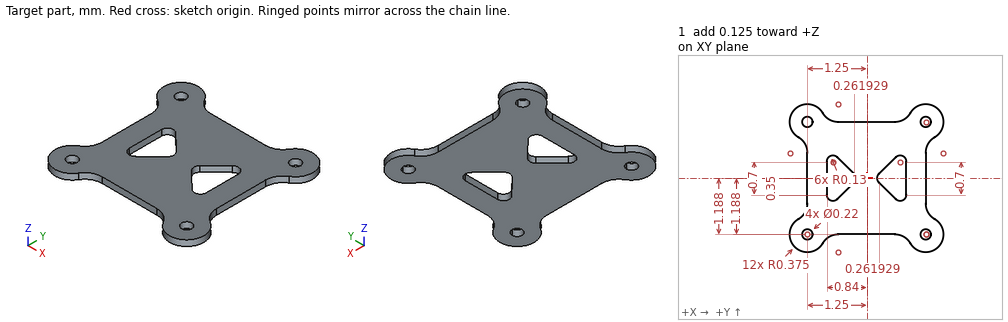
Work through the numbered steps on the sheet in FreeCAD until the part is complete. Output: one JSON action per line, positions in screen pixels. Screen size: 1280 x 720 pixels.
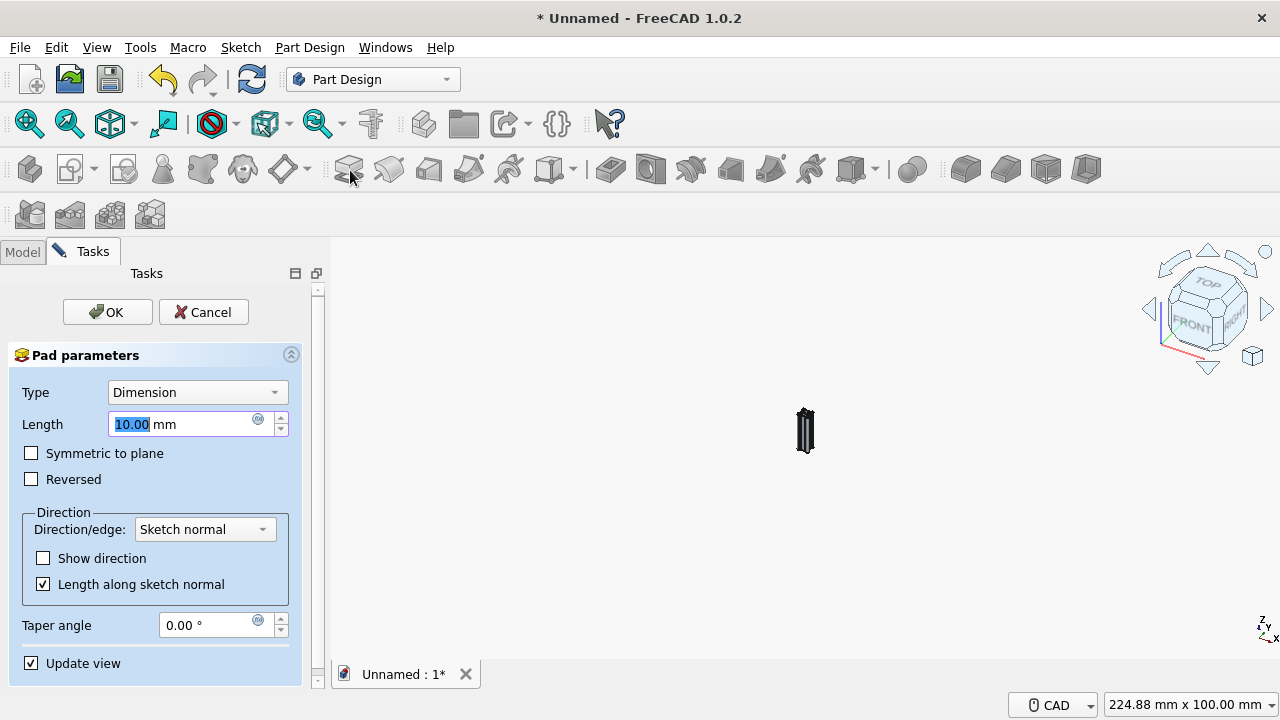
{"action": "type", "text": "0.125"}
{"action": "key", "text": "Tab"}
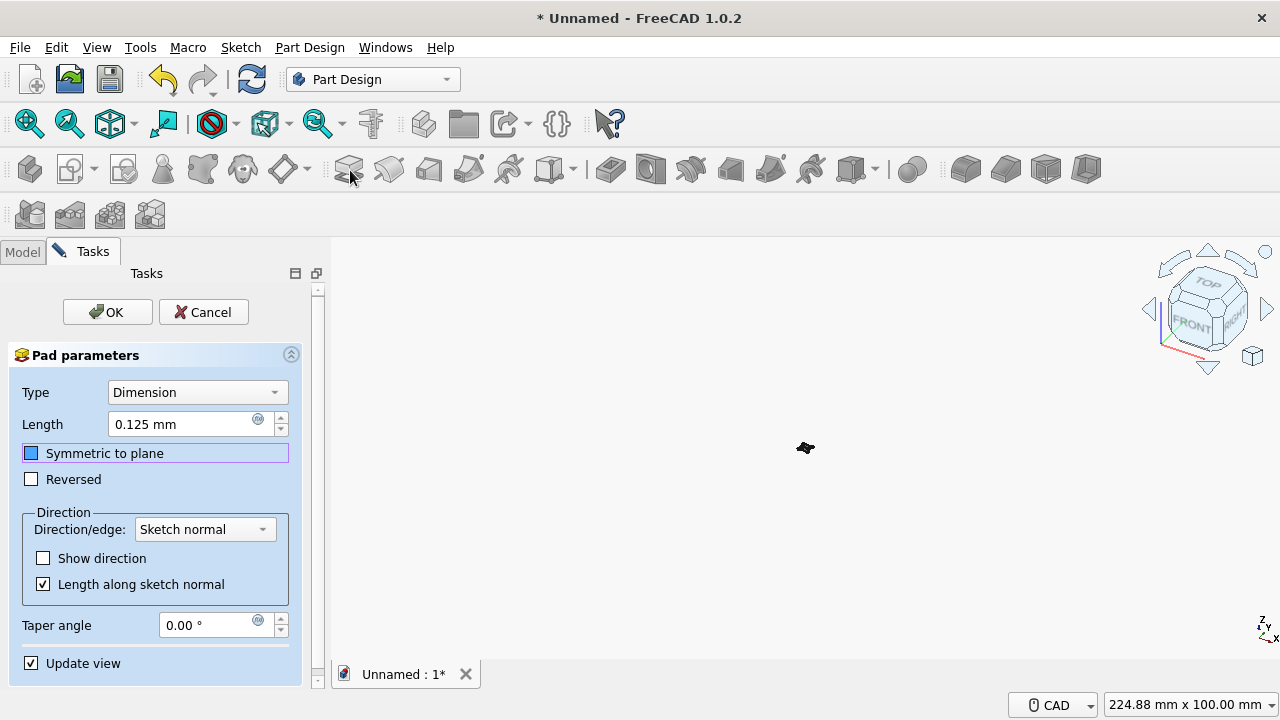
{"action": "left_click", "coordinate": [108, 312]}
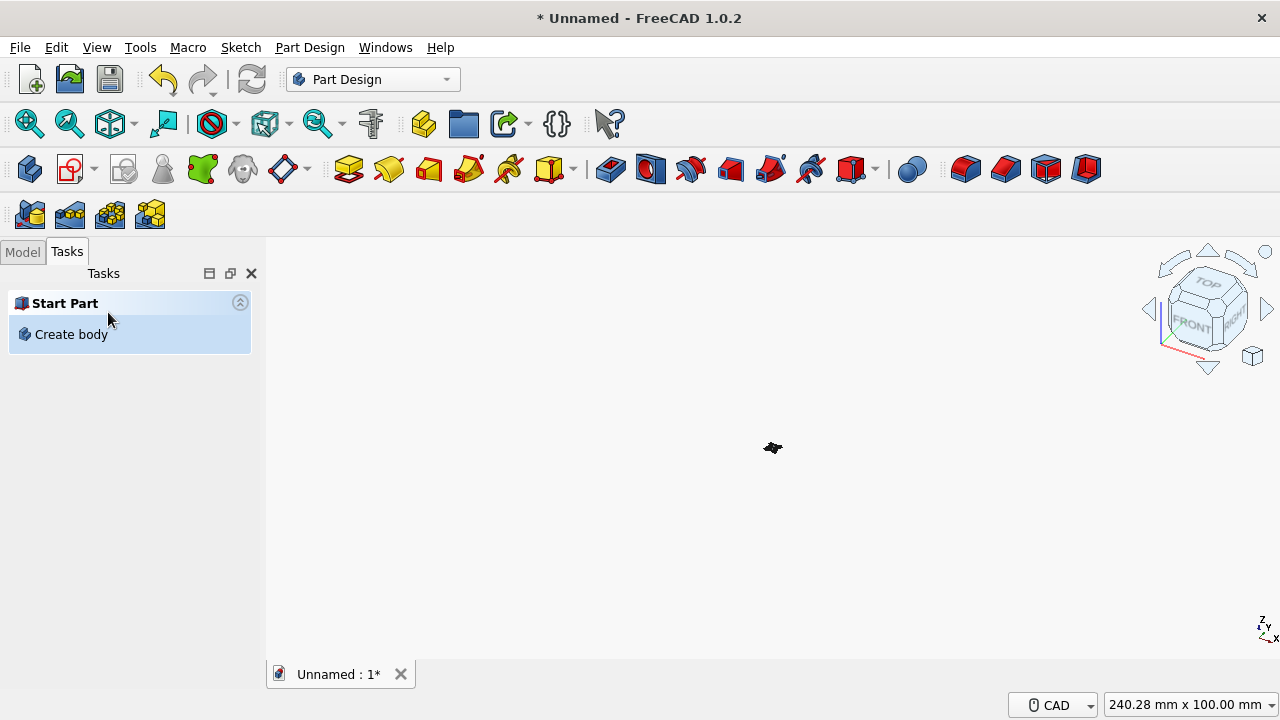
{"action": "key", "text": "0"}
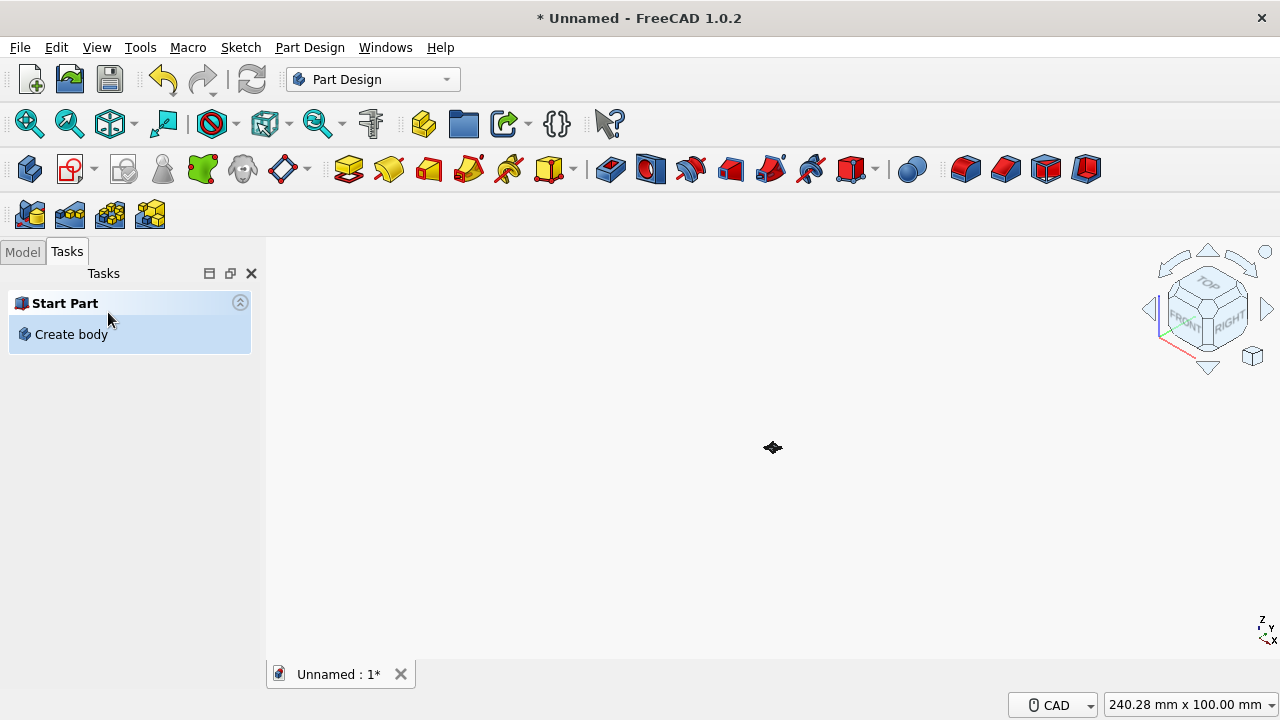
{"action": "left_click", "coordinate": [30, 124]}